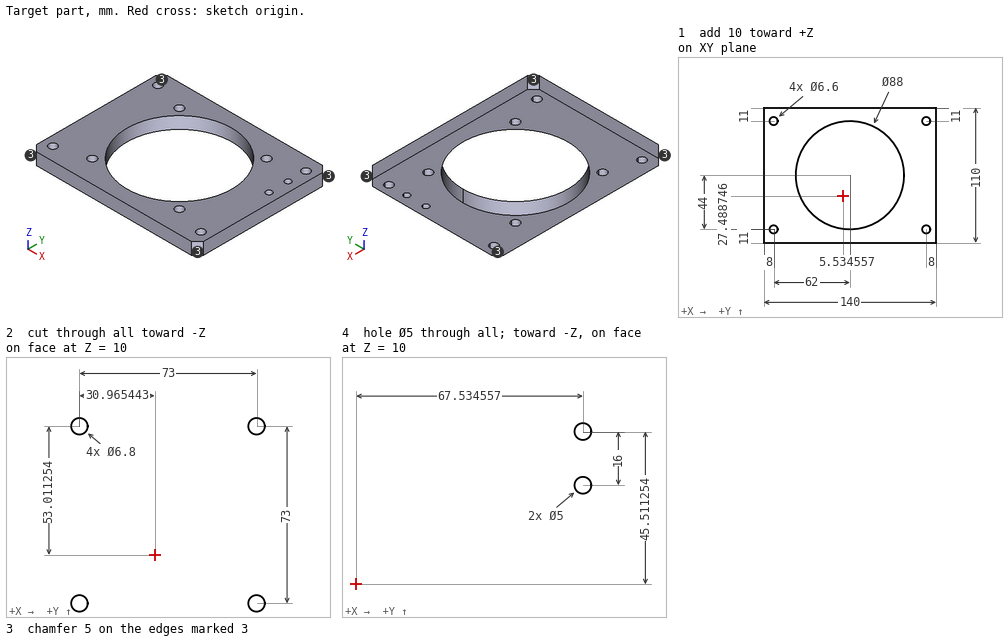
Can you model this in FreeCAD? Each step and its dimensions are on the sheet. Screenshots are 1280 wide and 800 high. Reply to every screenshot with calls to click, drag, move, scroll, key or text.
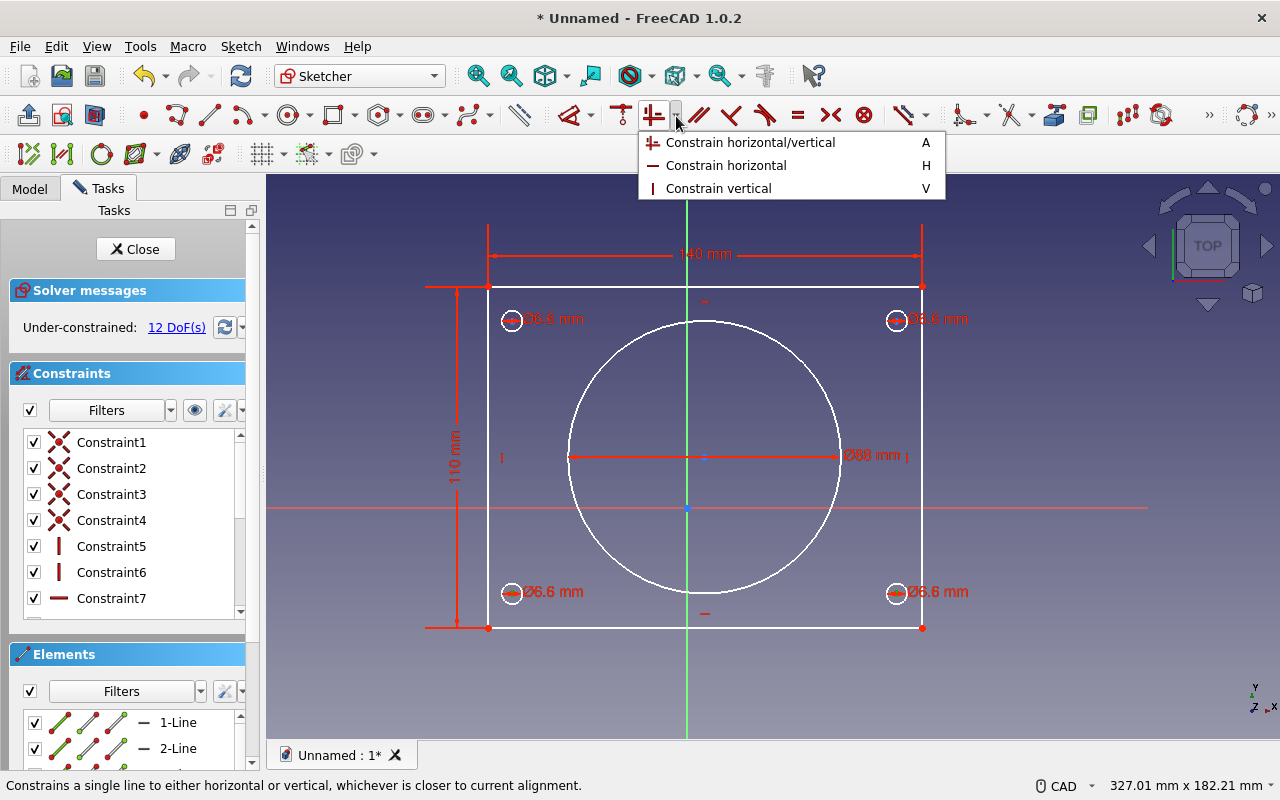
click(792, 166)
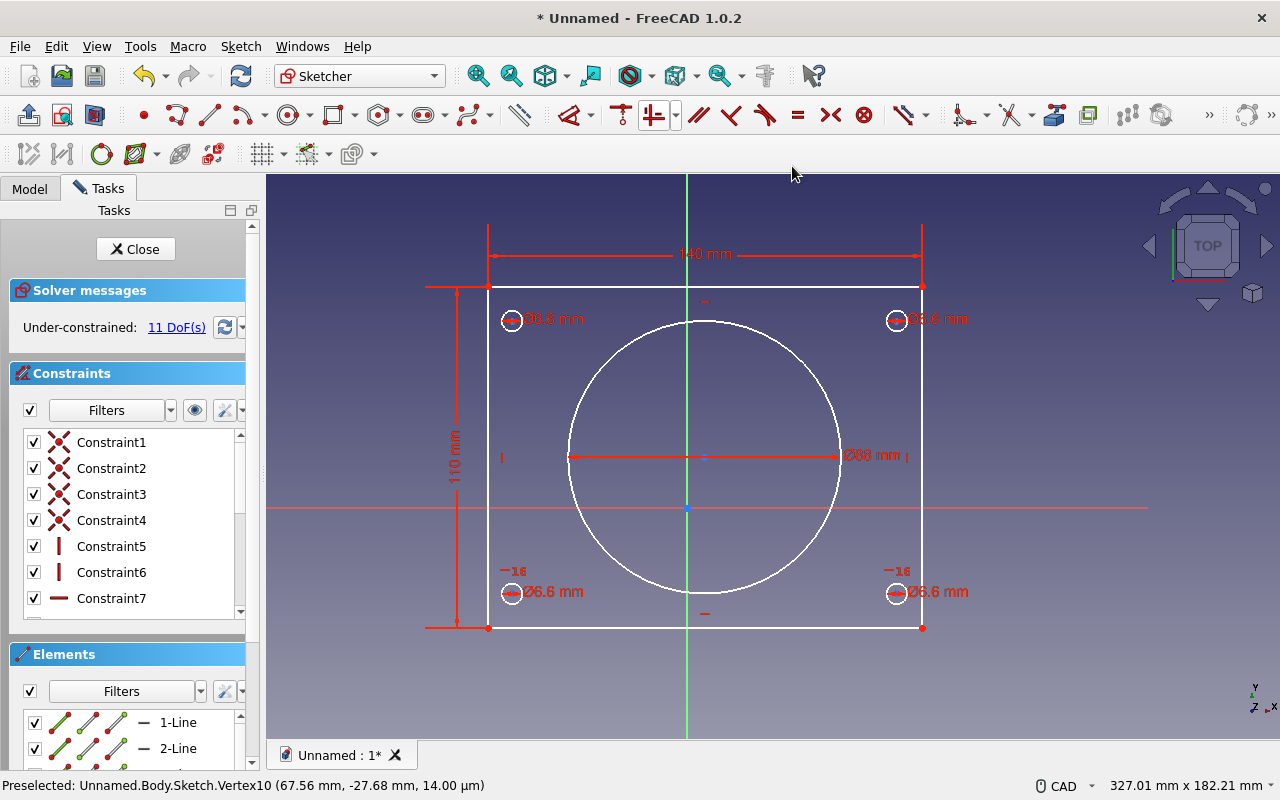
click(512, 594)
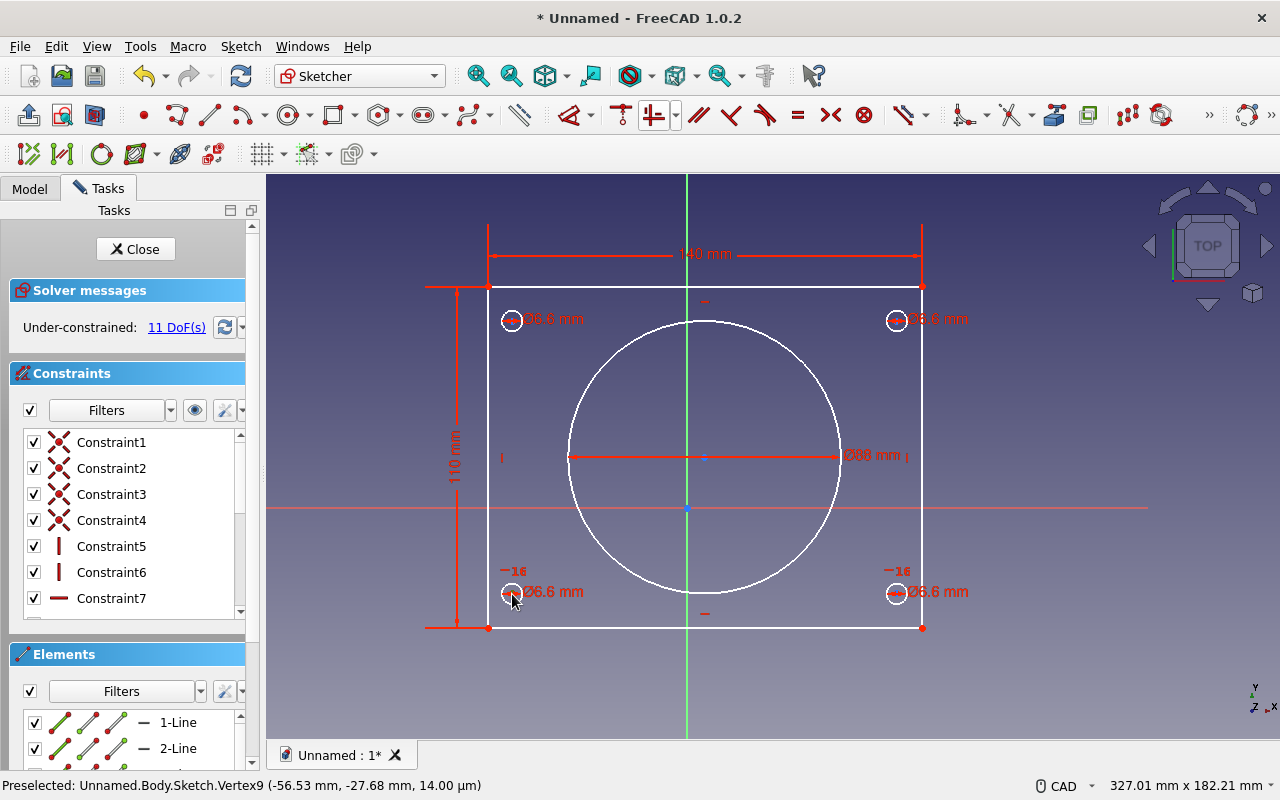
click(512, 321)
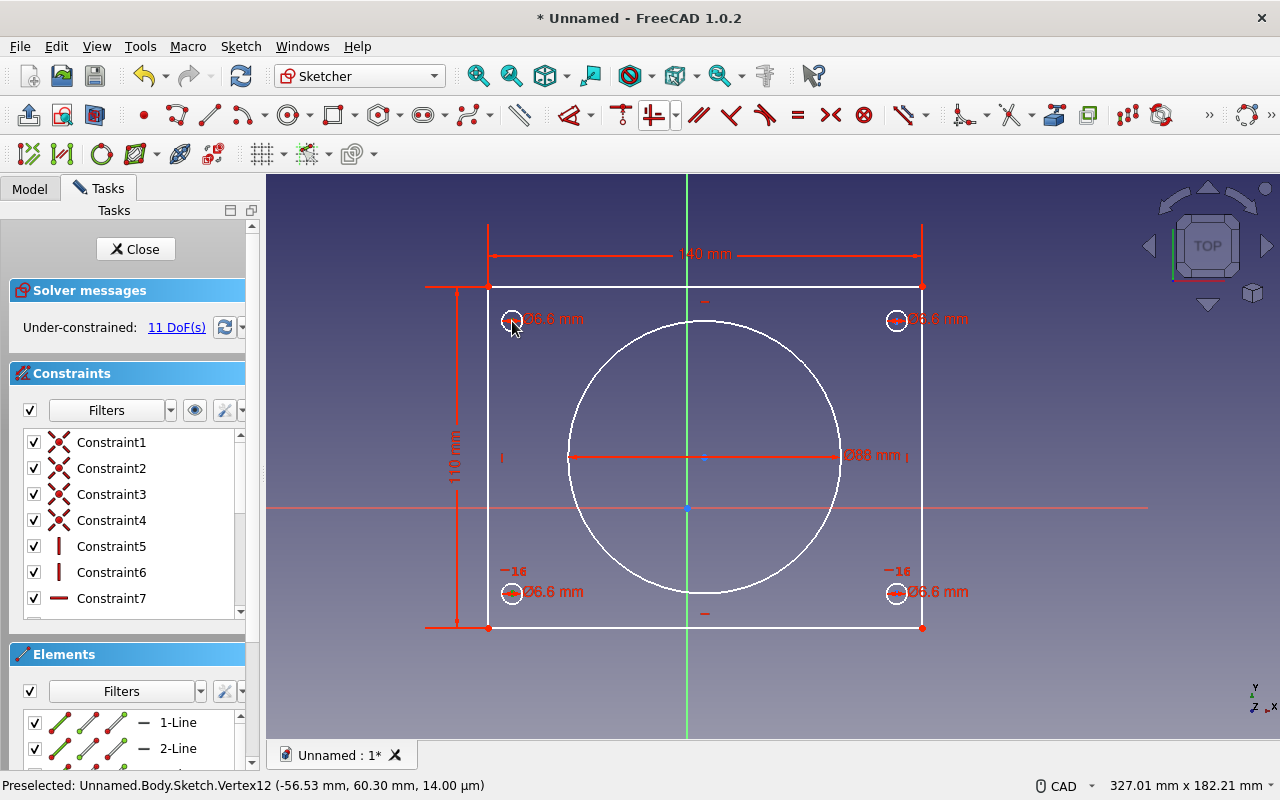
click(676, 116)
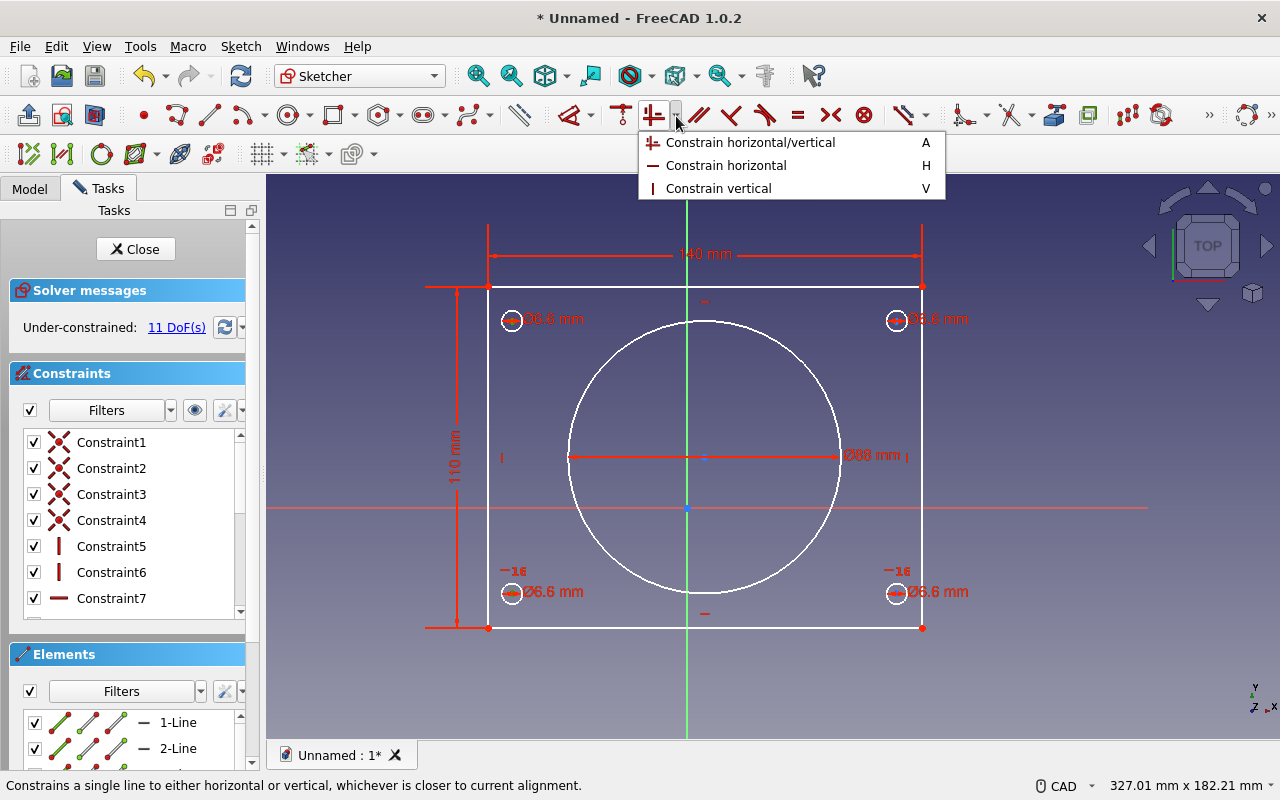
click(792, 188)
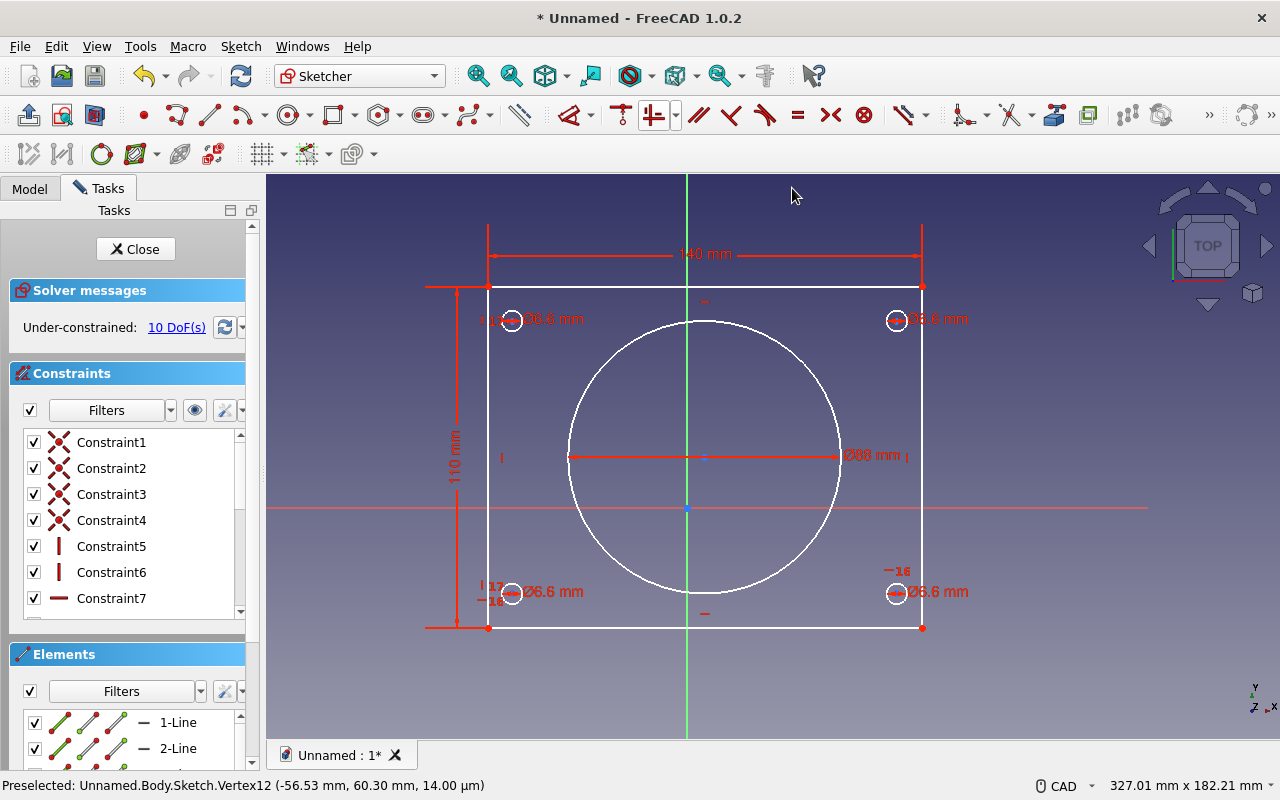
click(897, 594)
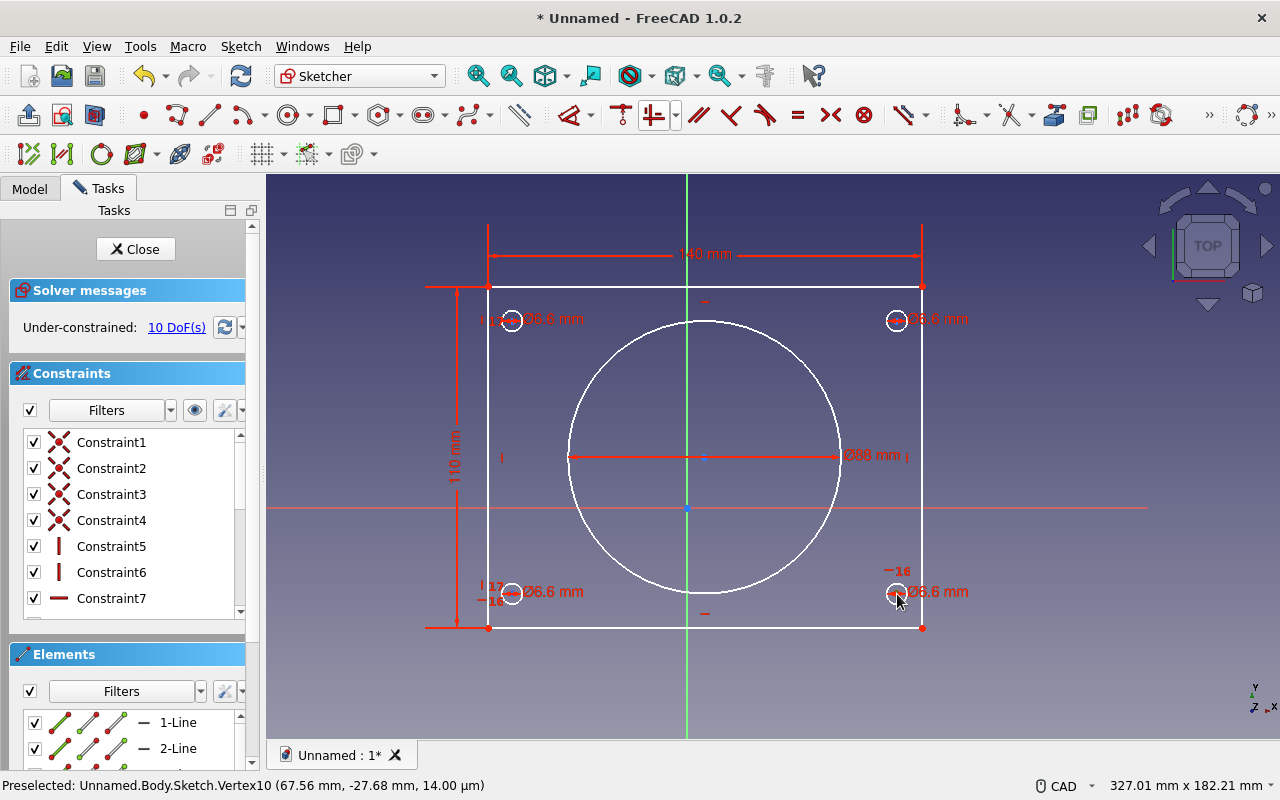
click(897, 321)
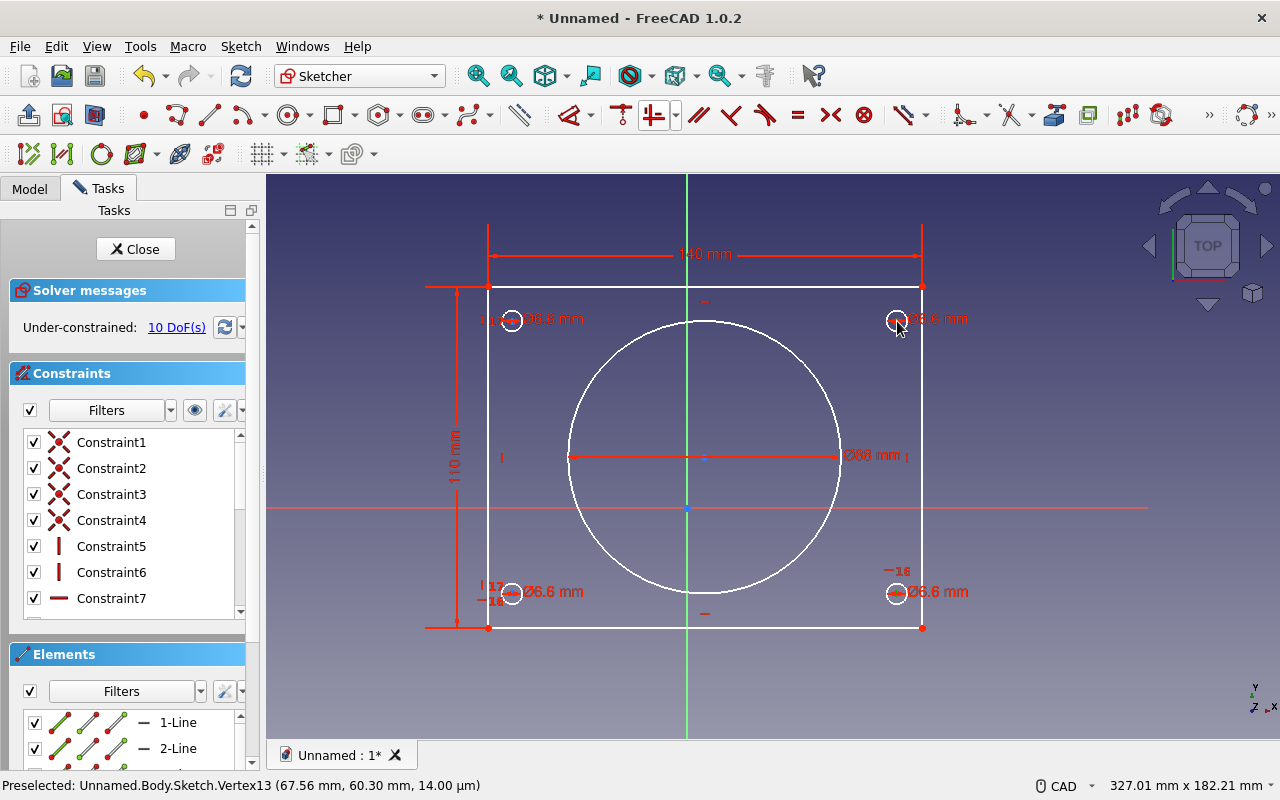
key(v)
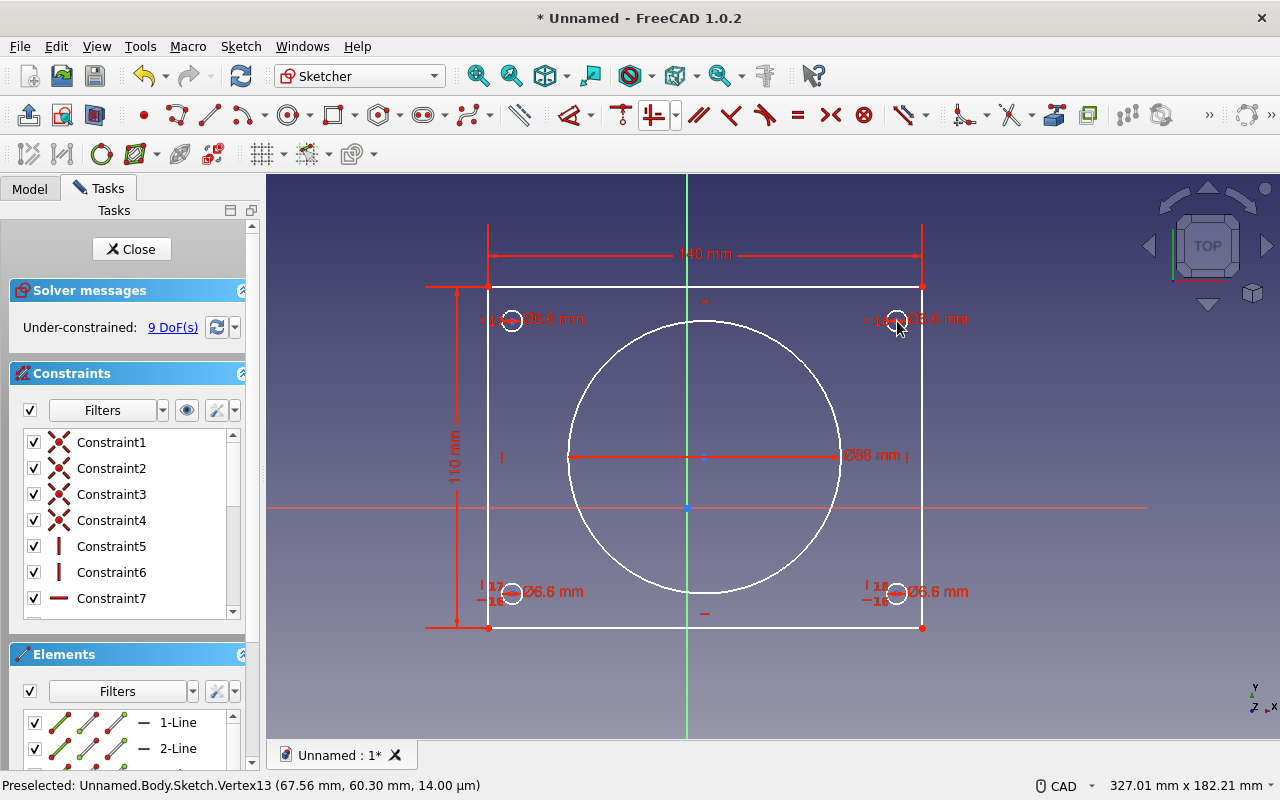
click(568, 116)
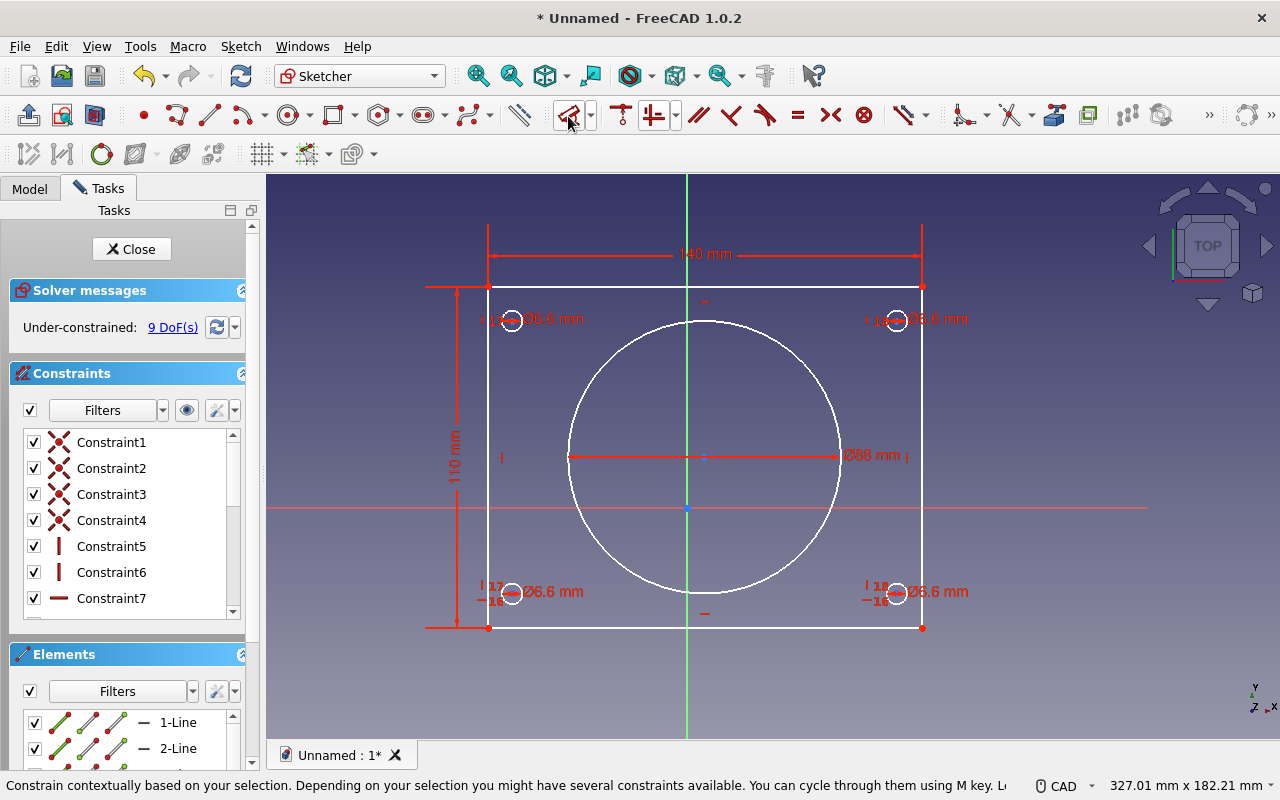
scroll(488, 628, up, 3)